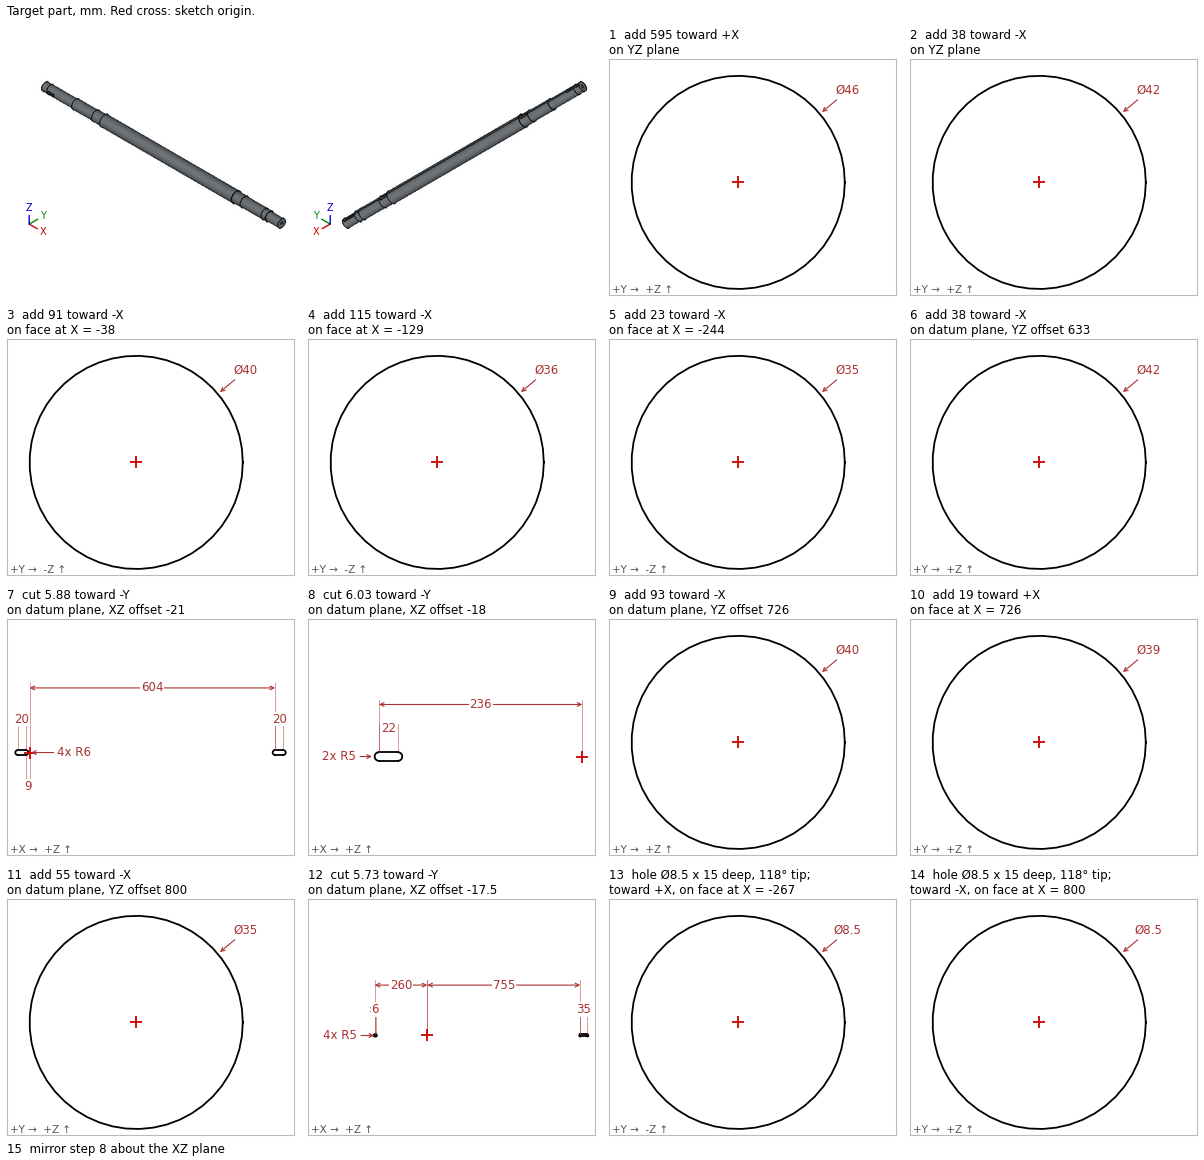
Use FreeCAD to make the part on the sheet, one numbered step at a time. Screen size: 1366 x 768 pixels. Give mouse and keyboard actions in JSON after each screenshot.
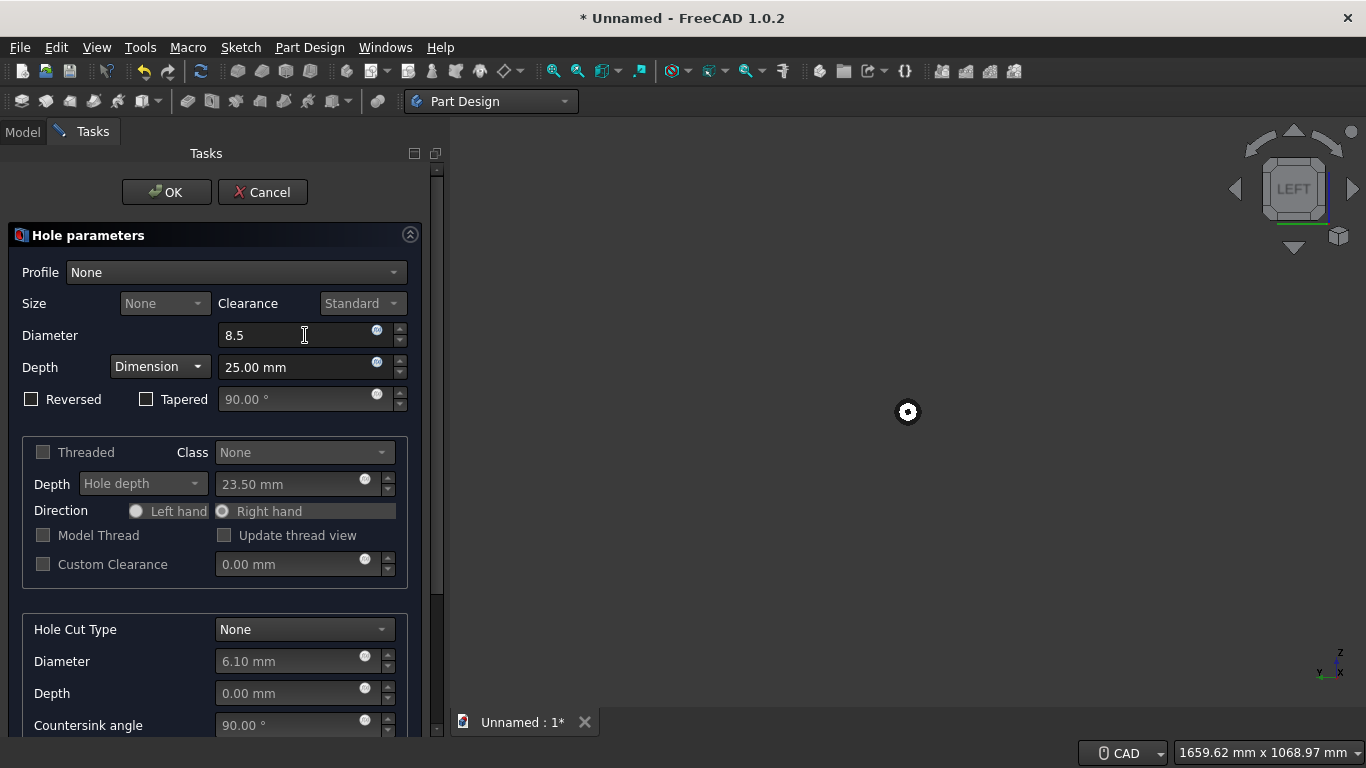
{"action": "triple_click", "coordinate": [305, 367]}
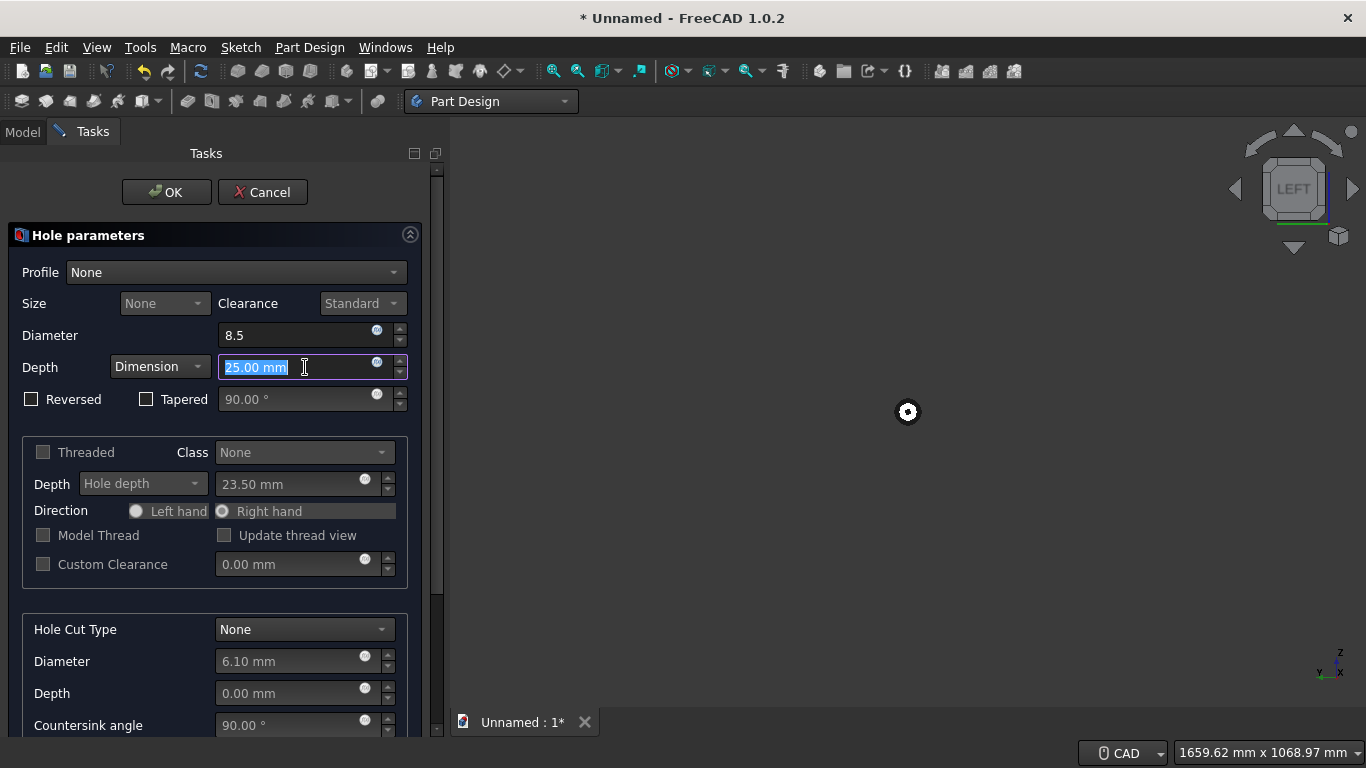
{"action": "type", "text": "15"}
{"action": "key", "text": "Tab"}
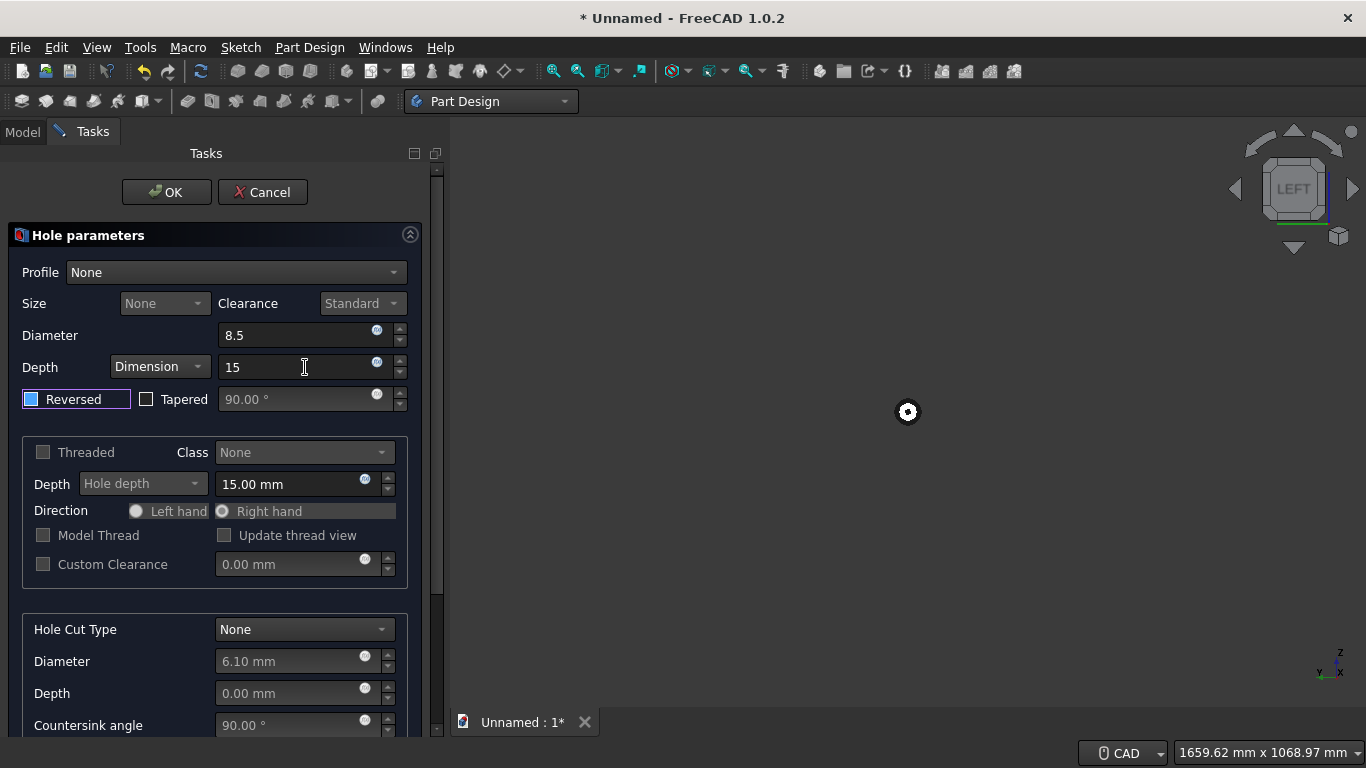
{"action": "left_click", "coordinate": [167, 192]}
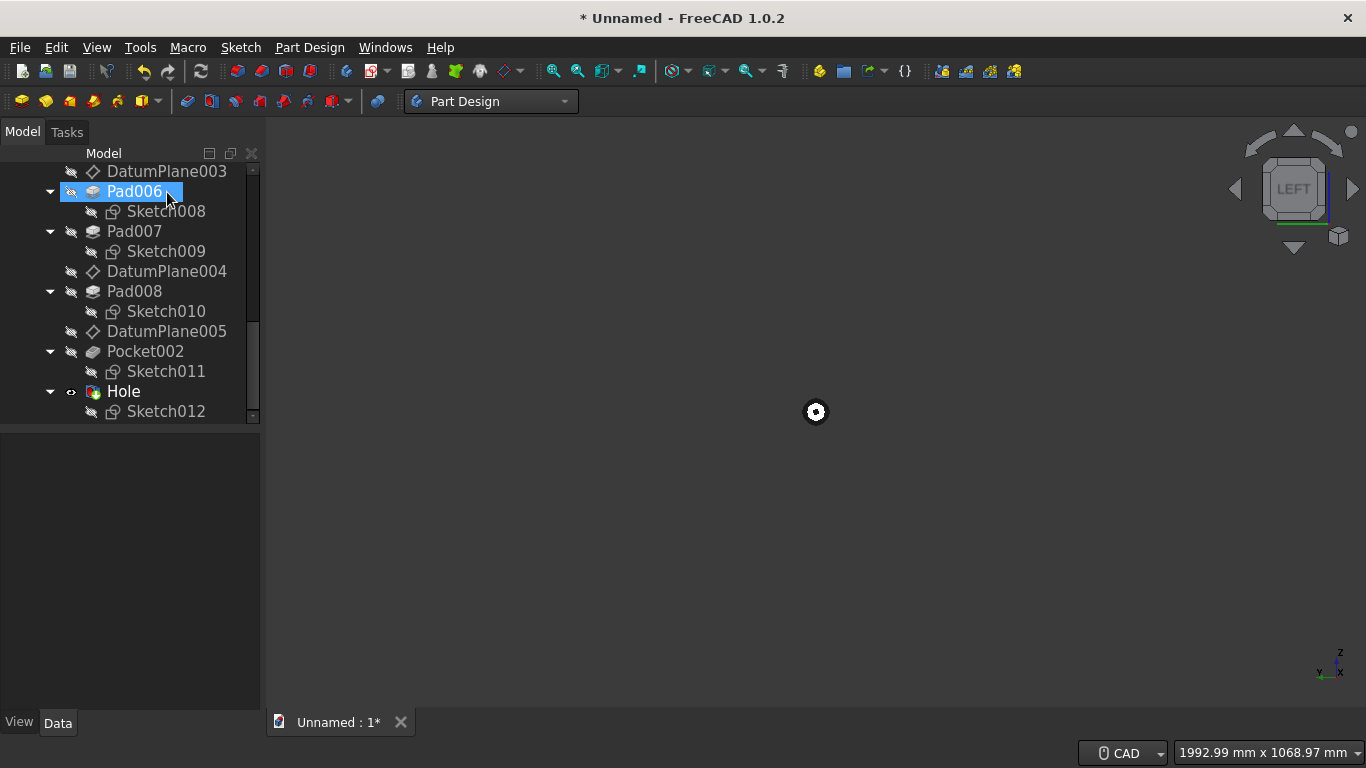
{"action": "key", "text": "v f"}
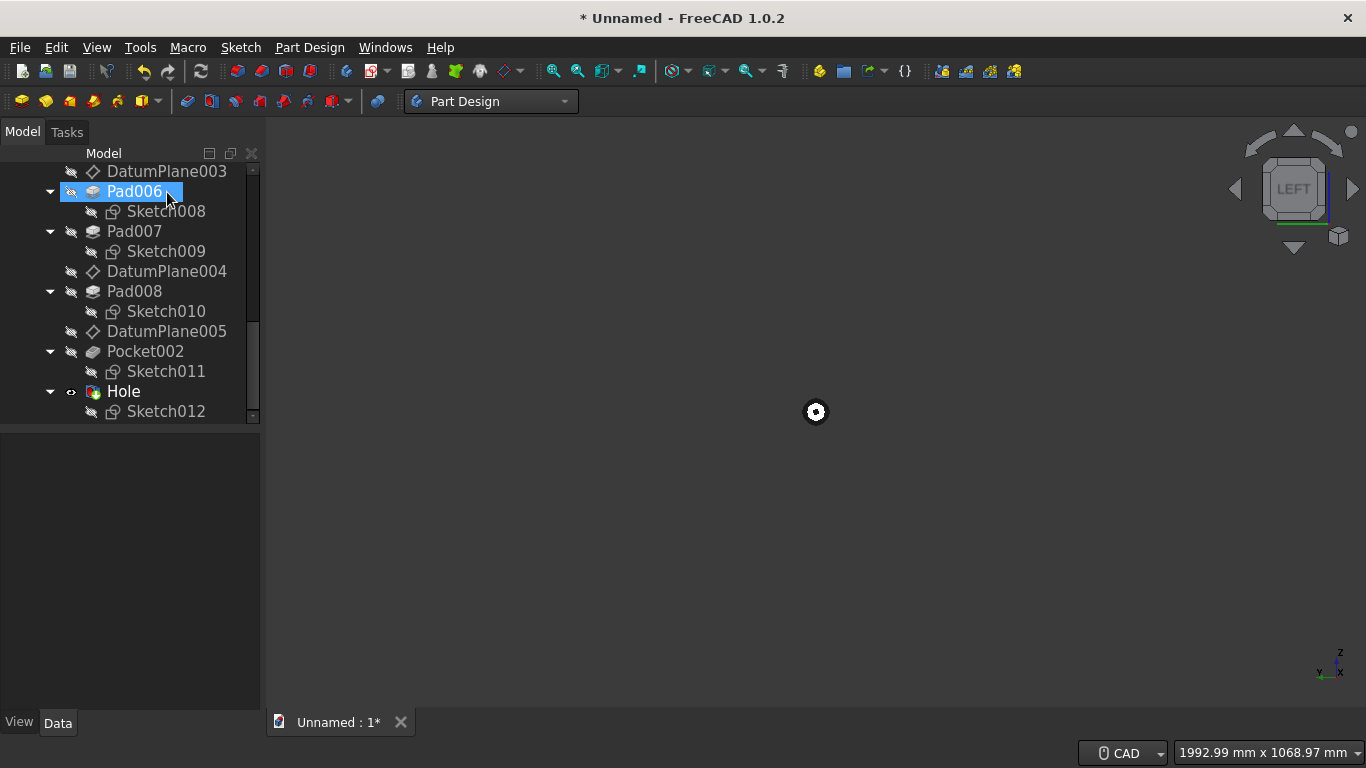
{"action": "key", "text": "0"}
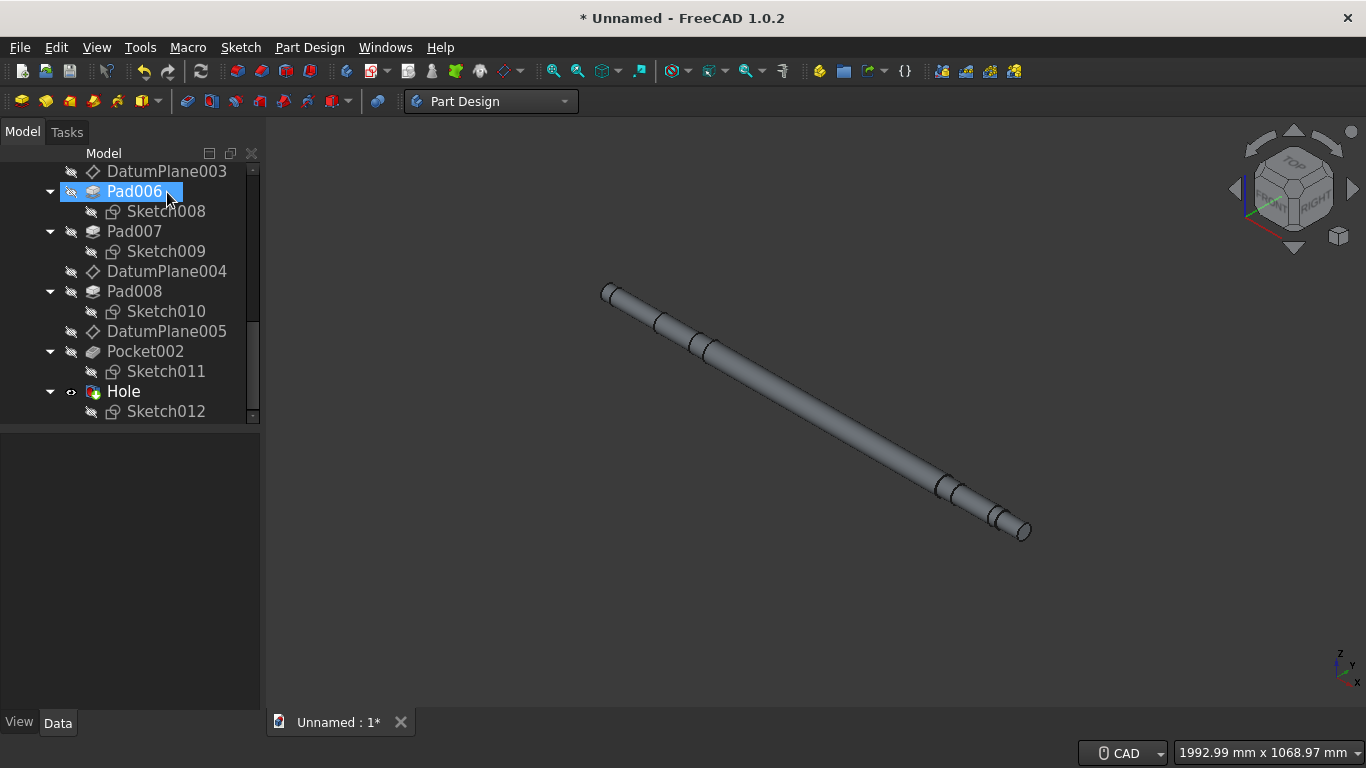
{"action": "key", "text": "3"}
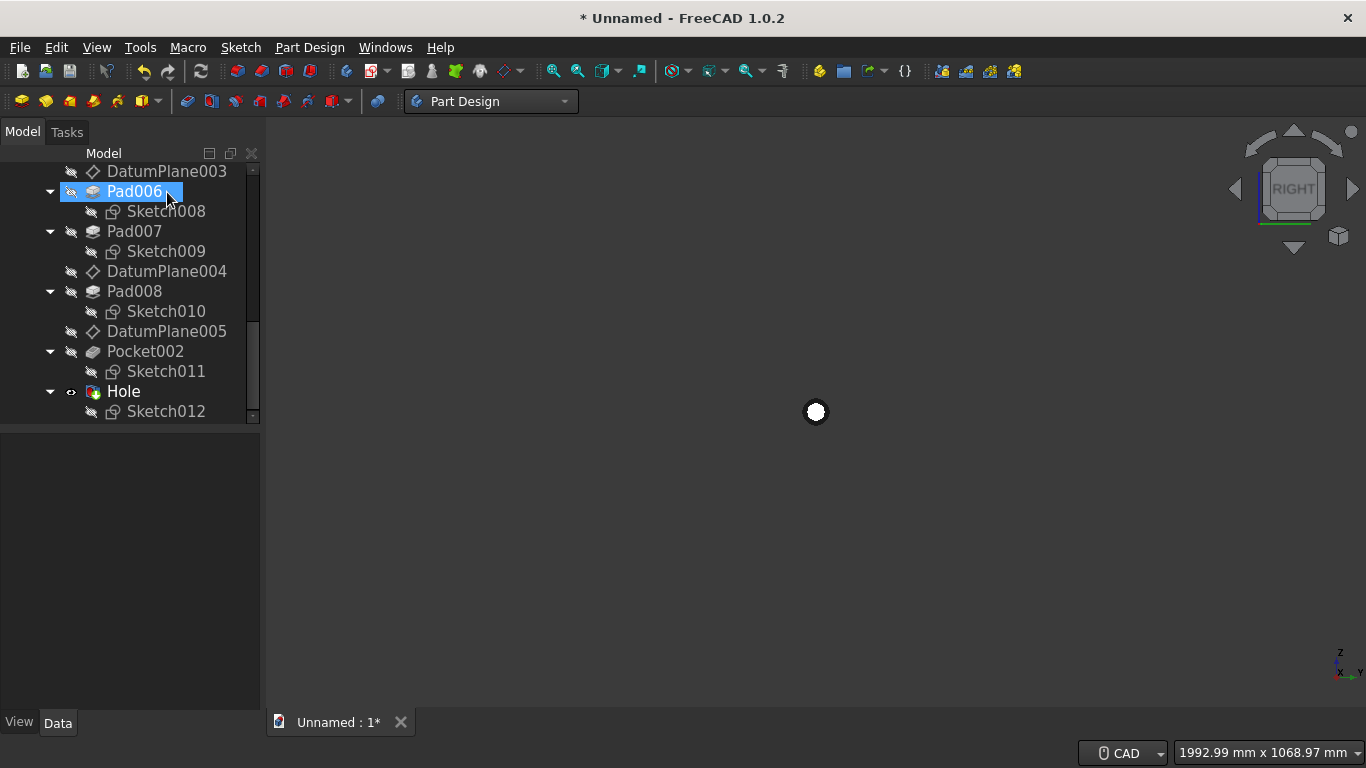
{"action": "key", "text": "v f"}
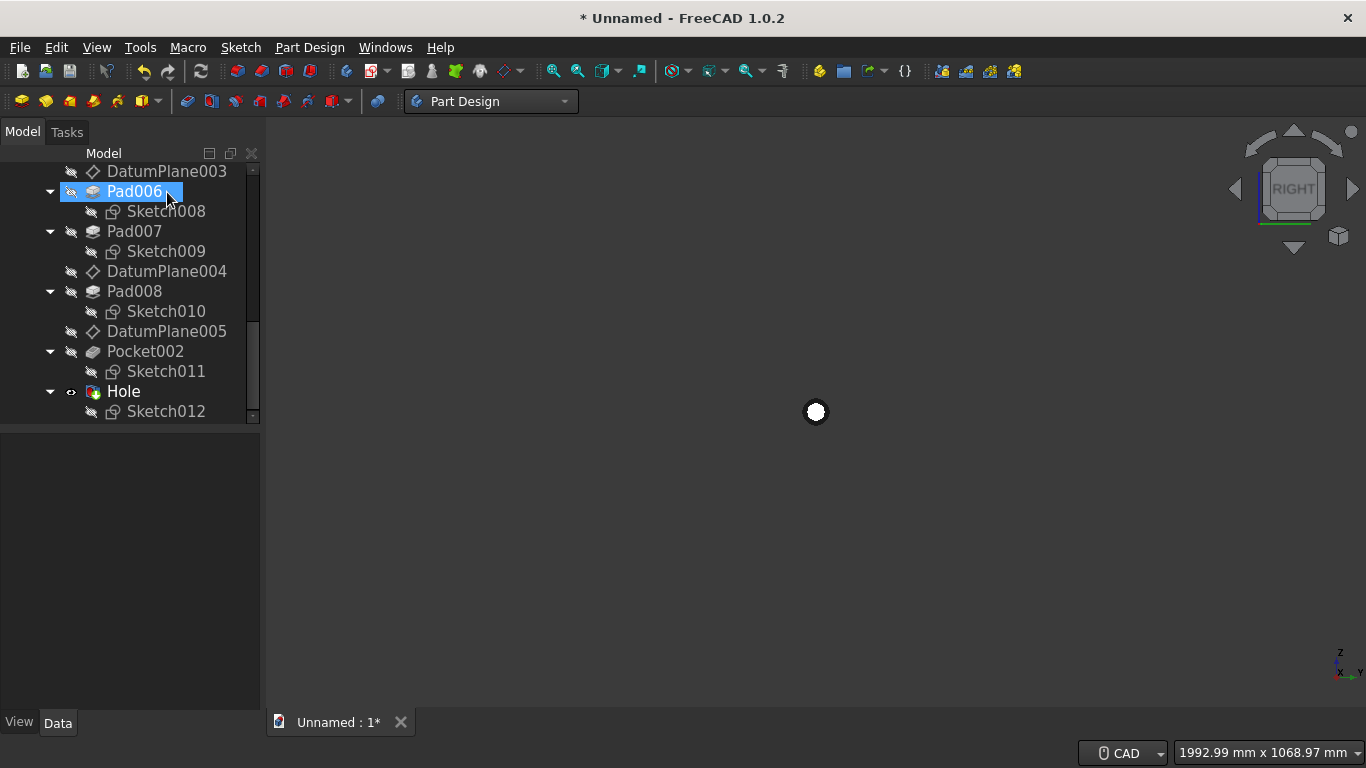
{"action": "left_click", "coordinate": [816, 411]}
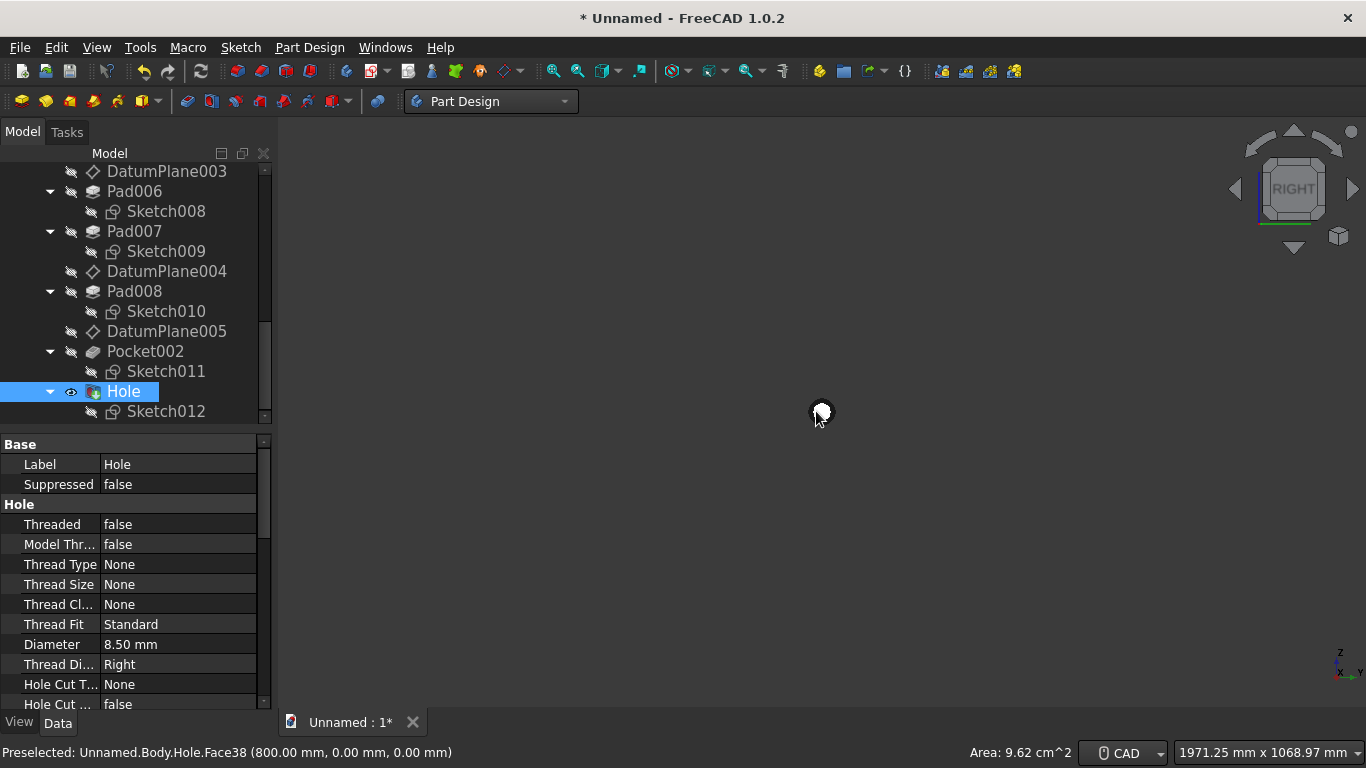
{"action": "left_click", "coordinate": [372, 72]}